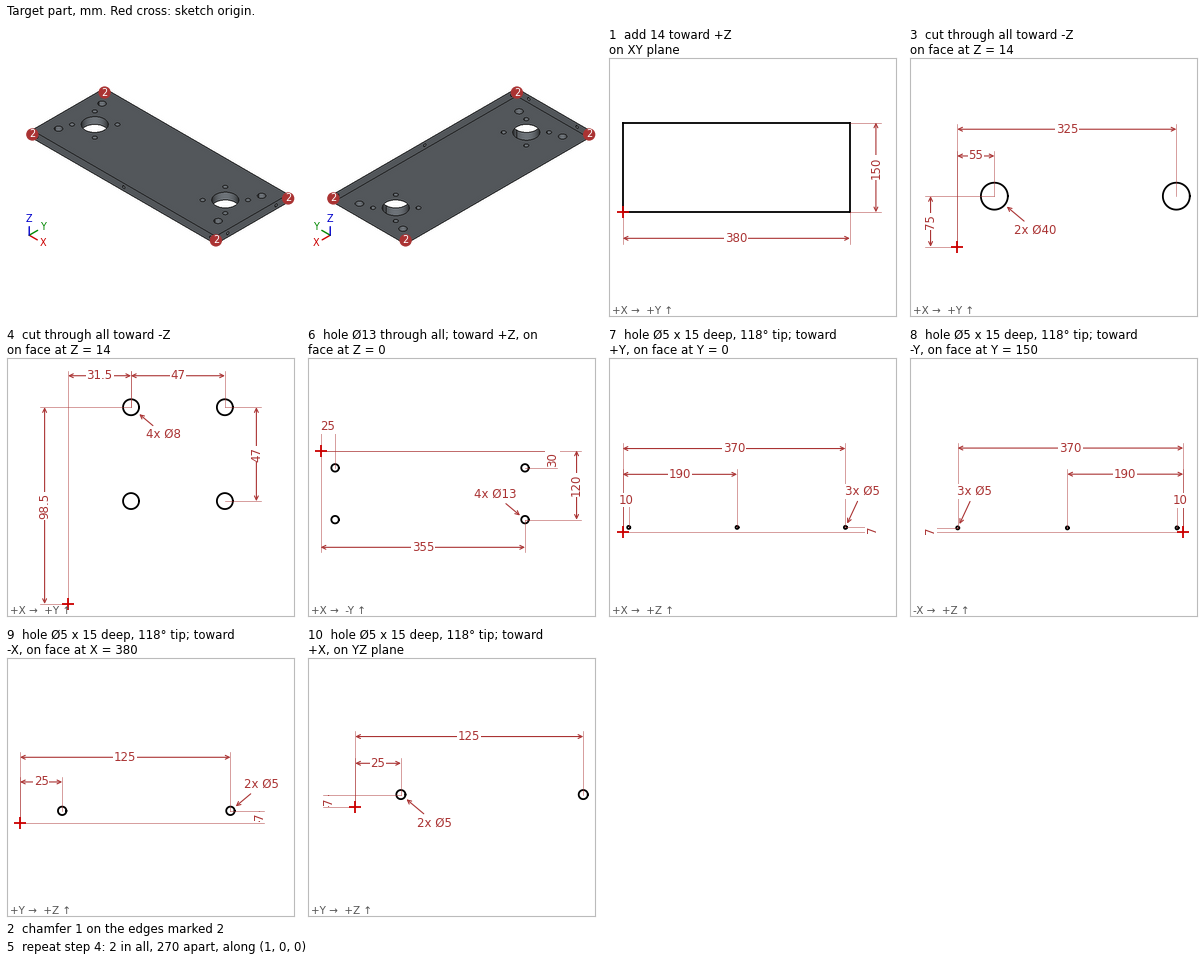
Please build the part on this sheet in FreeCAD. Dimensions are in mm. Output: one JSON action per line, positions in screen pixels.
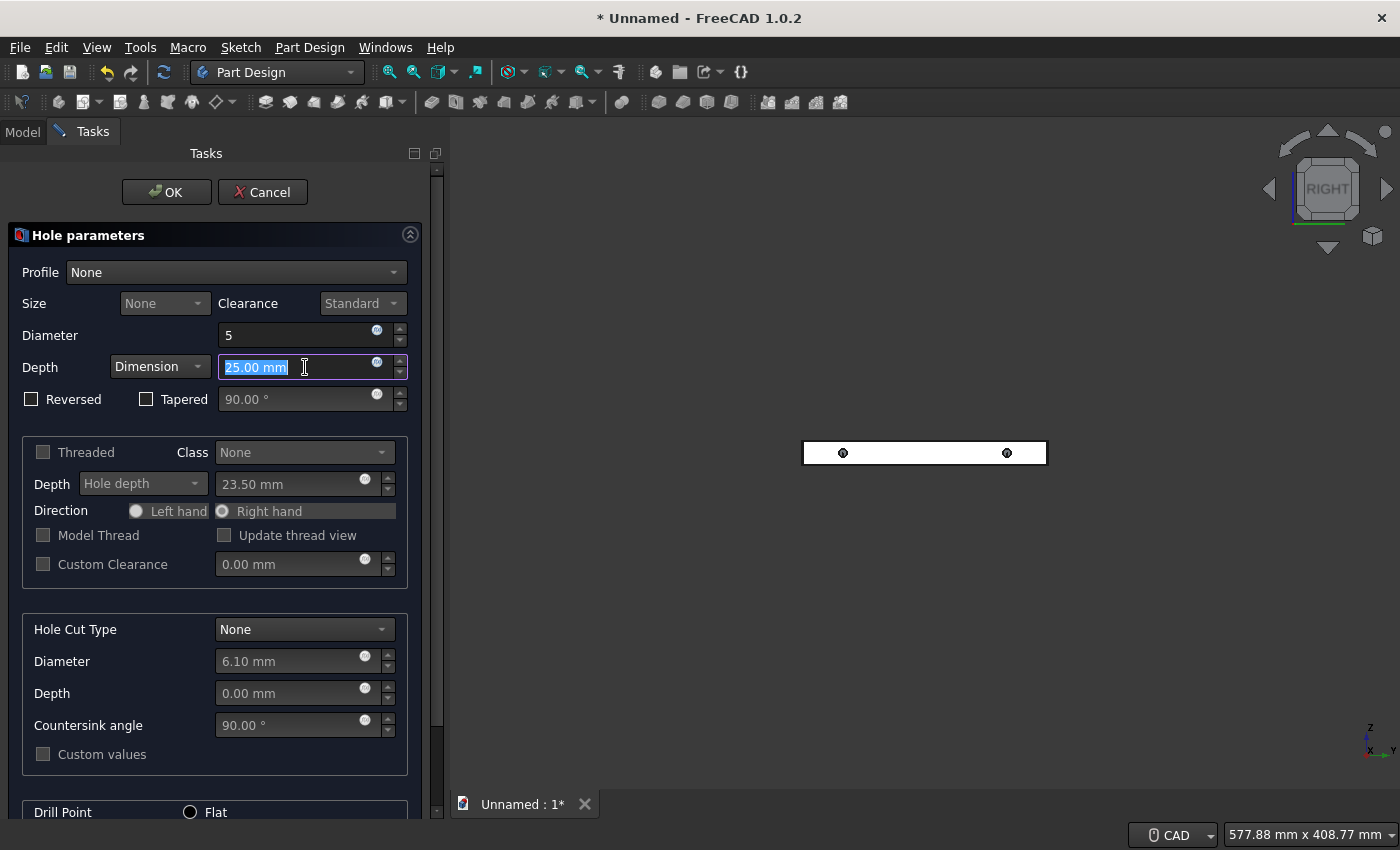
{"action": "type", "text": "15"}
{"action": "key", "text": "Tab"}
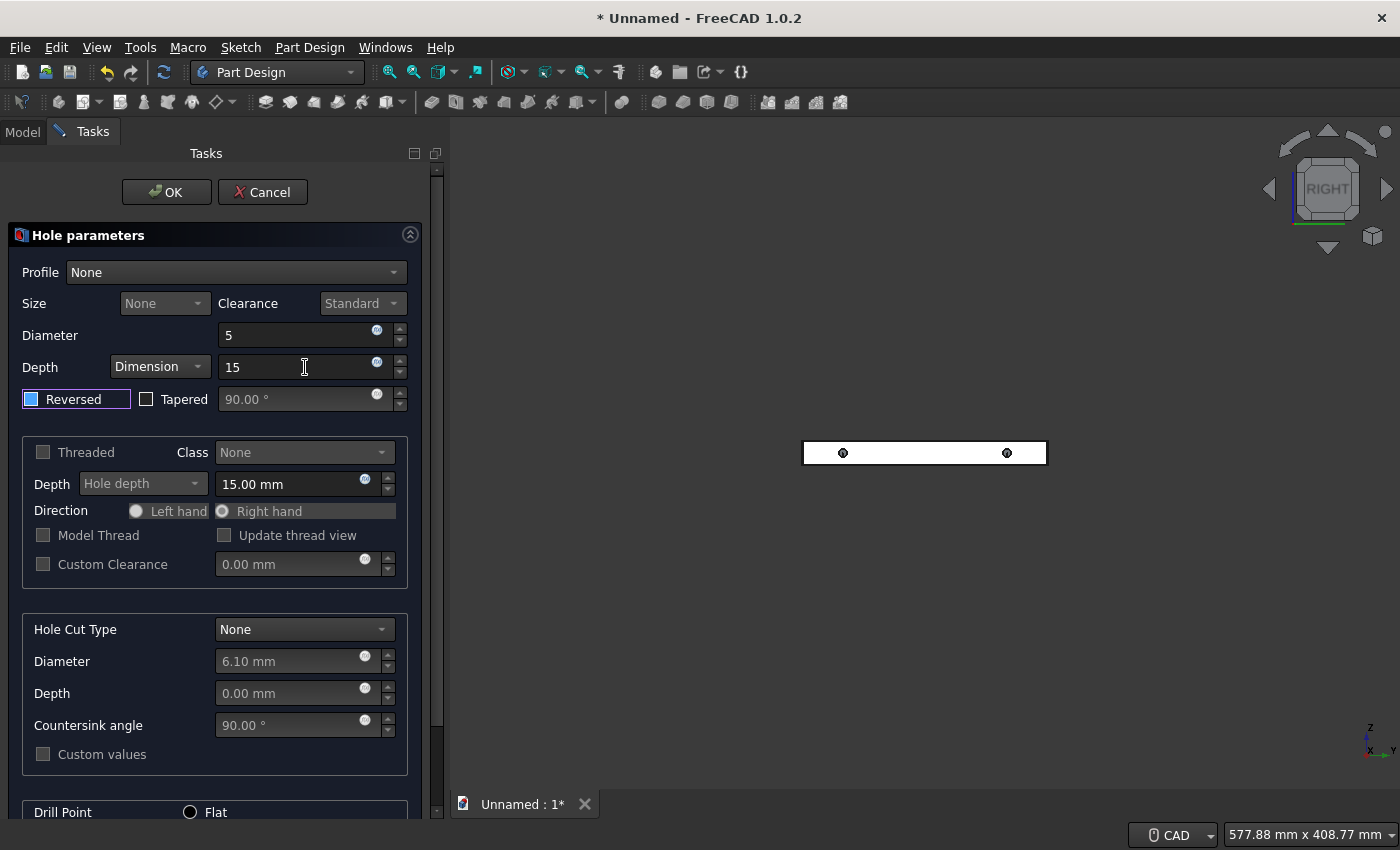
{"action": "left_click", "coordinate": [30, 399]}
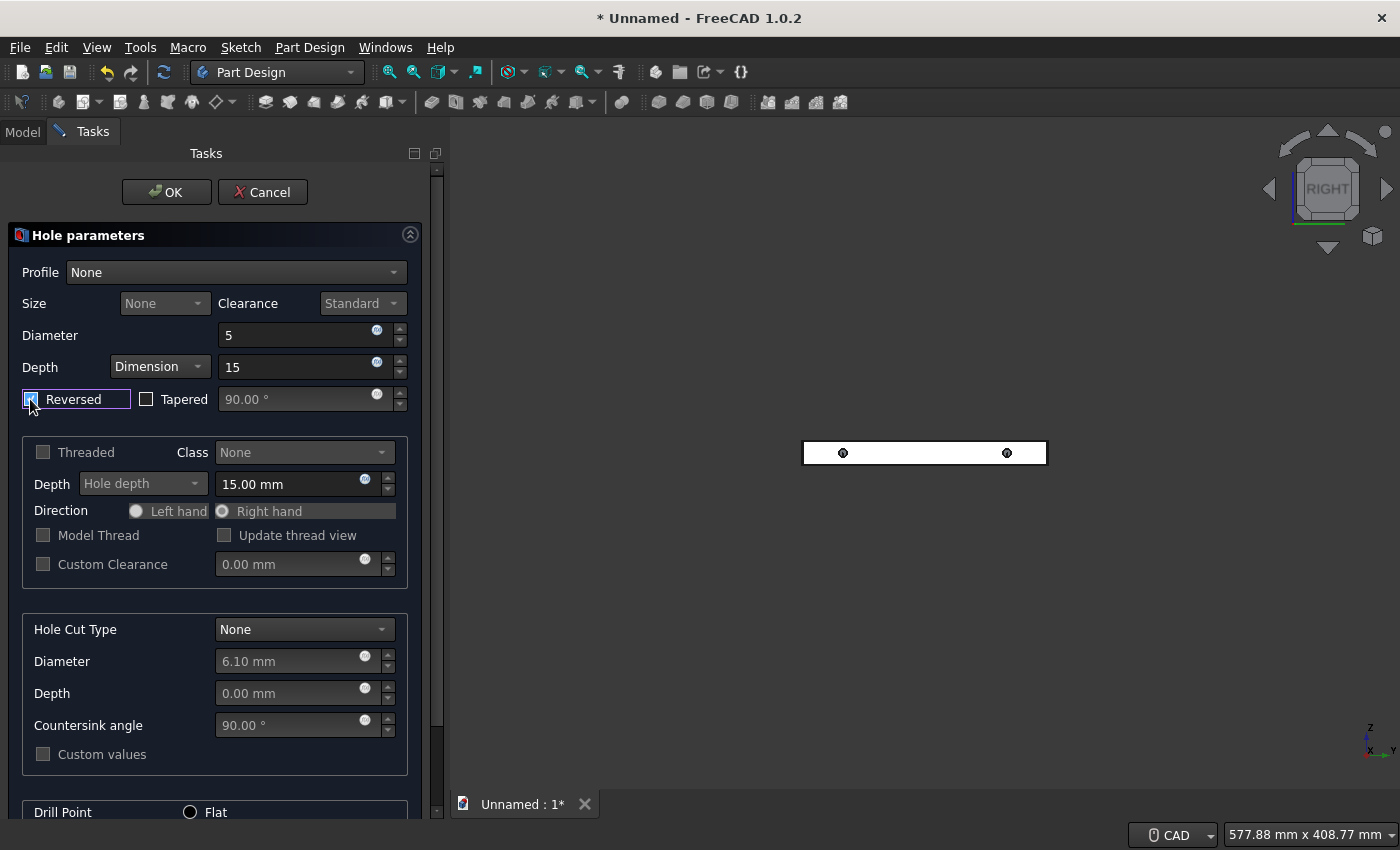
{"action": "left_click", "coordinate": [167, 192]}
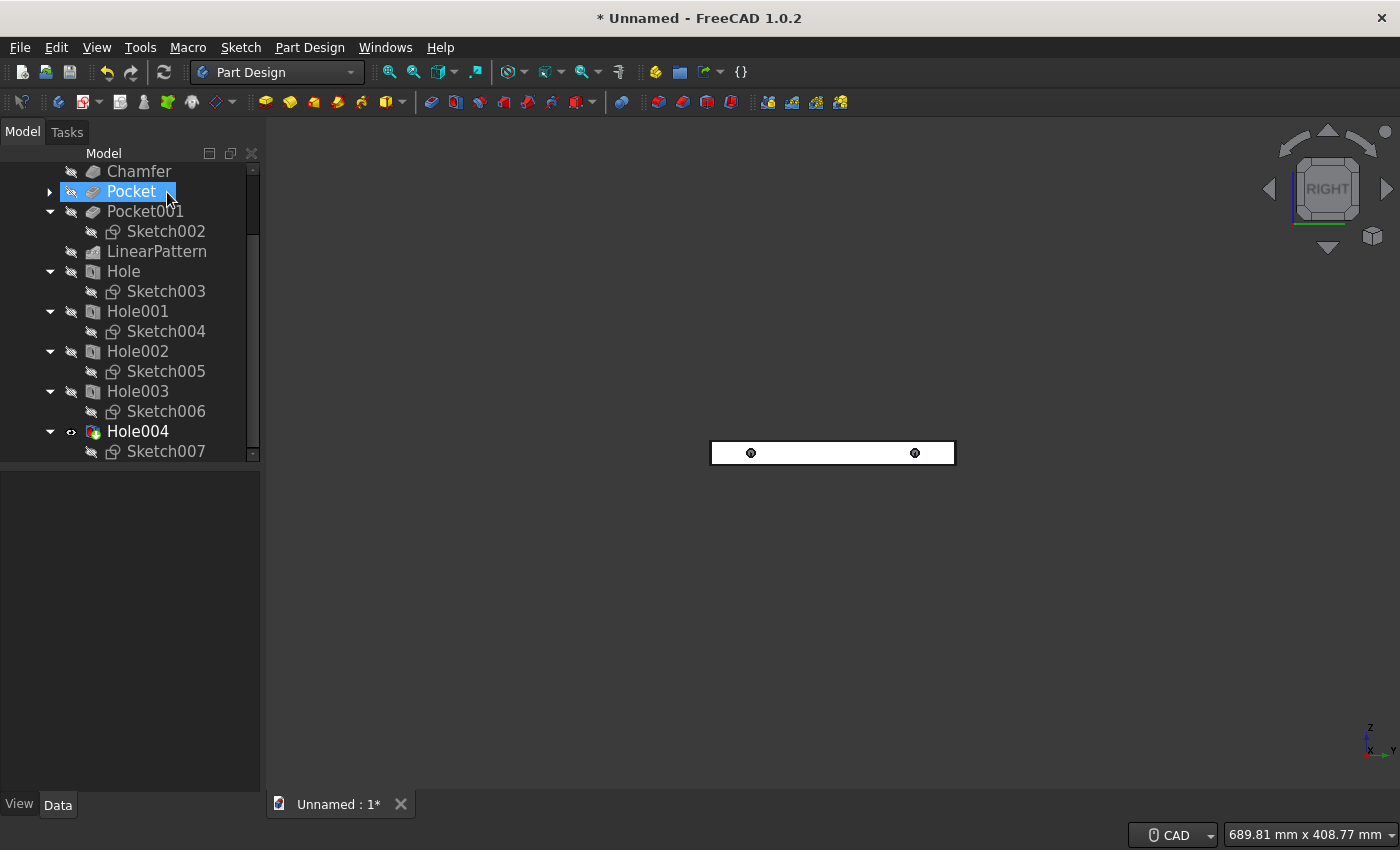
{"action": "key", "text": "0"}